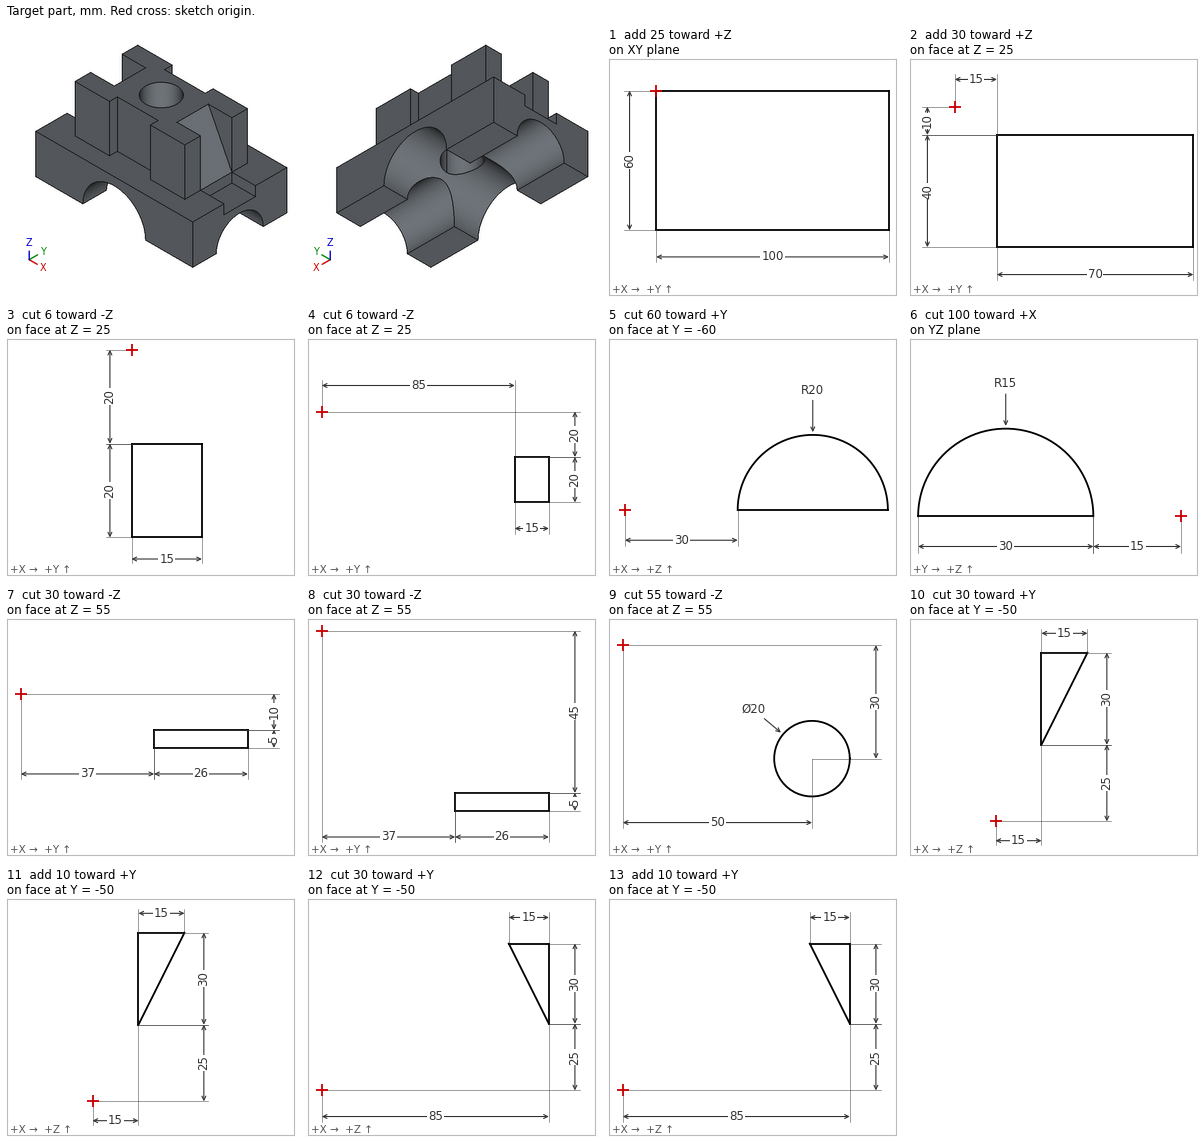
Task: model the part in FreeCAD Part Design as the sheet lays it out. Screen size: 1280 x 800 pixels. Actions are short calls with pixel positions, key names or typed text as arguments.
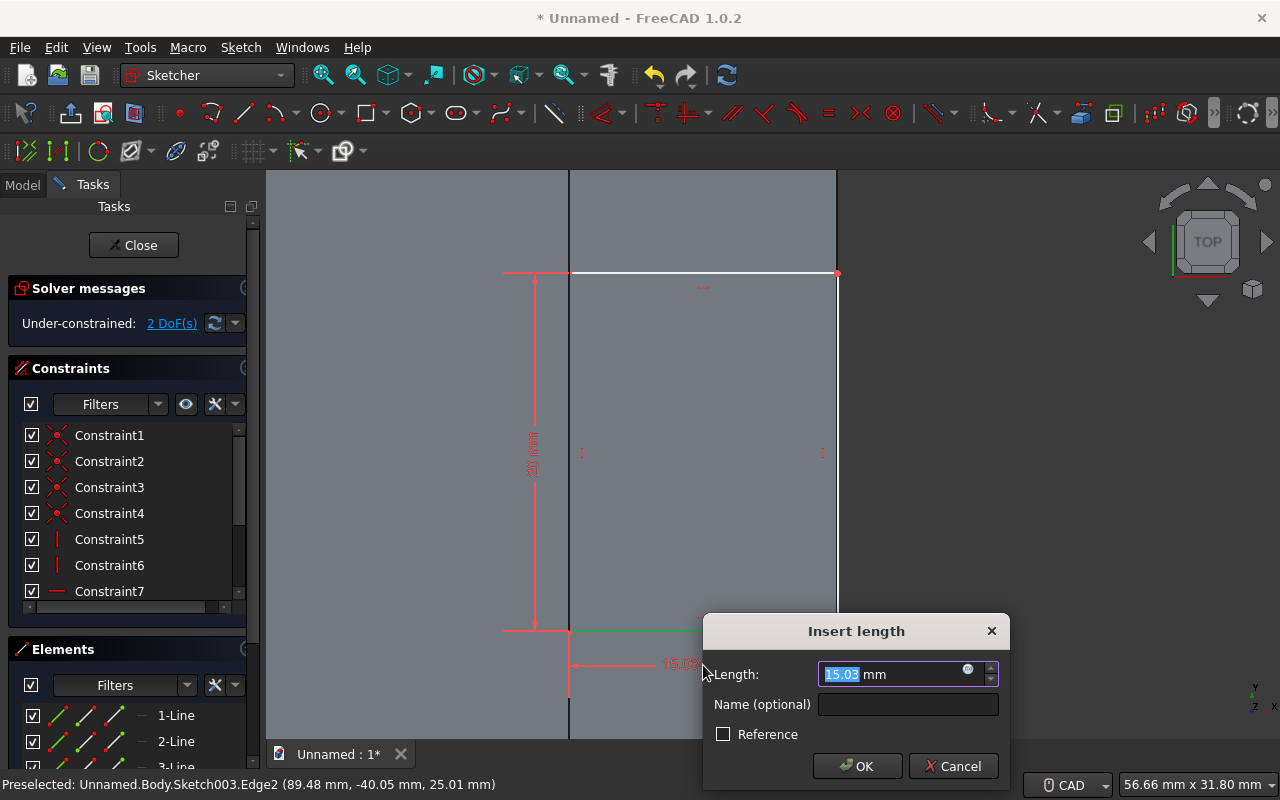
text(15)
key(Return)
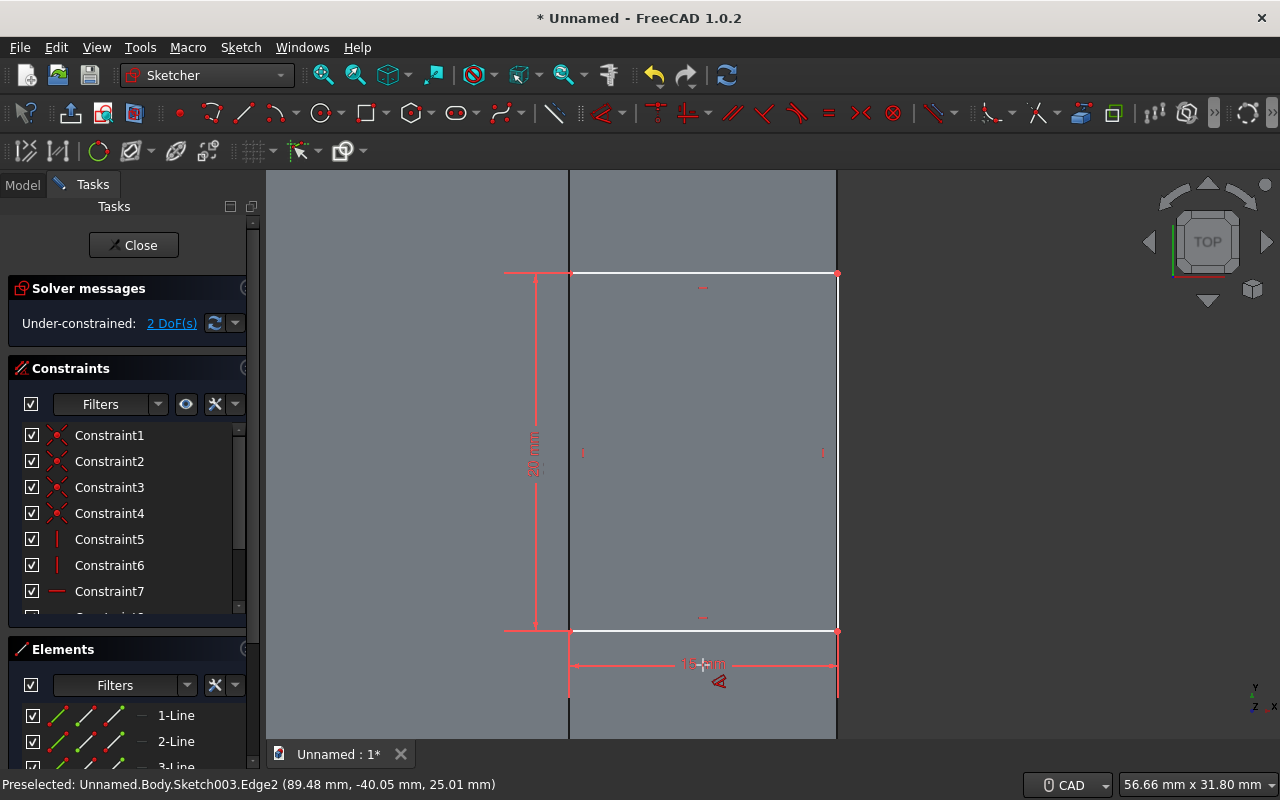
click(569, 273)
click(432, 307)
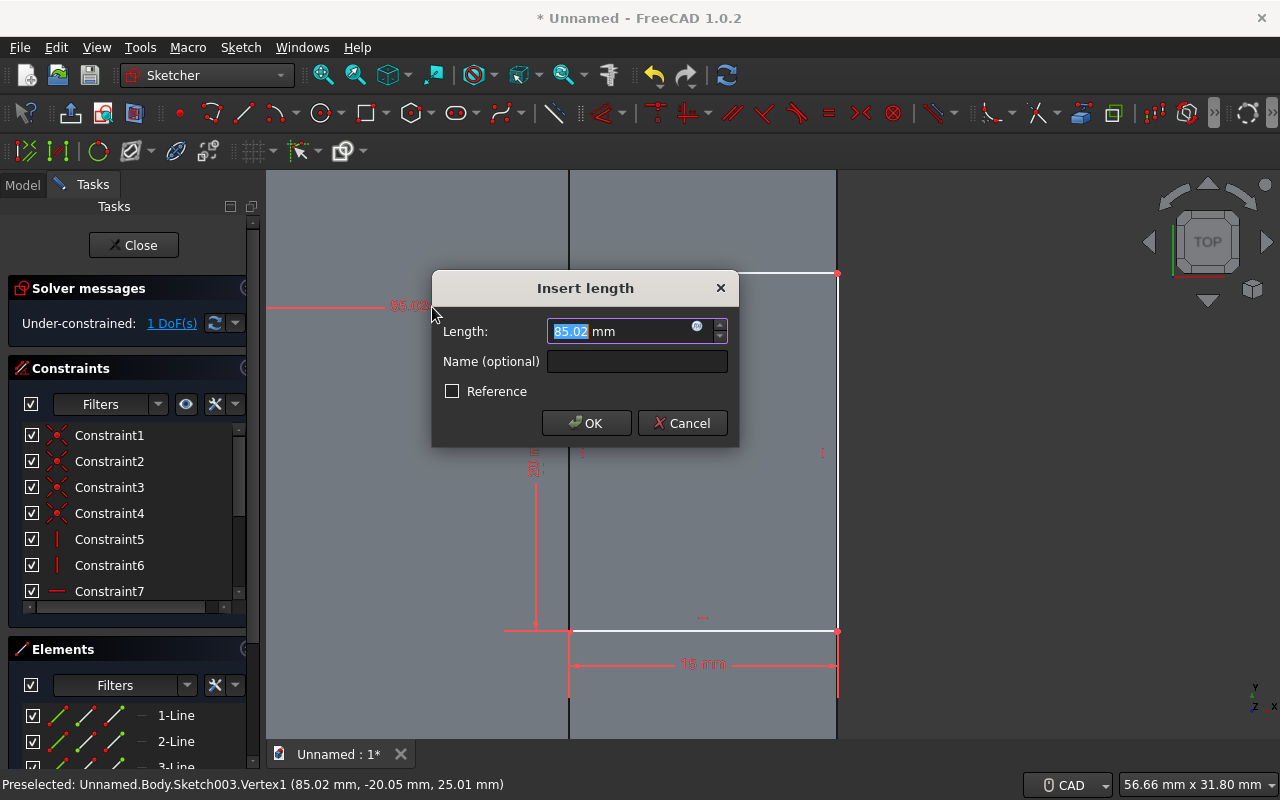
text(85)
key(Return)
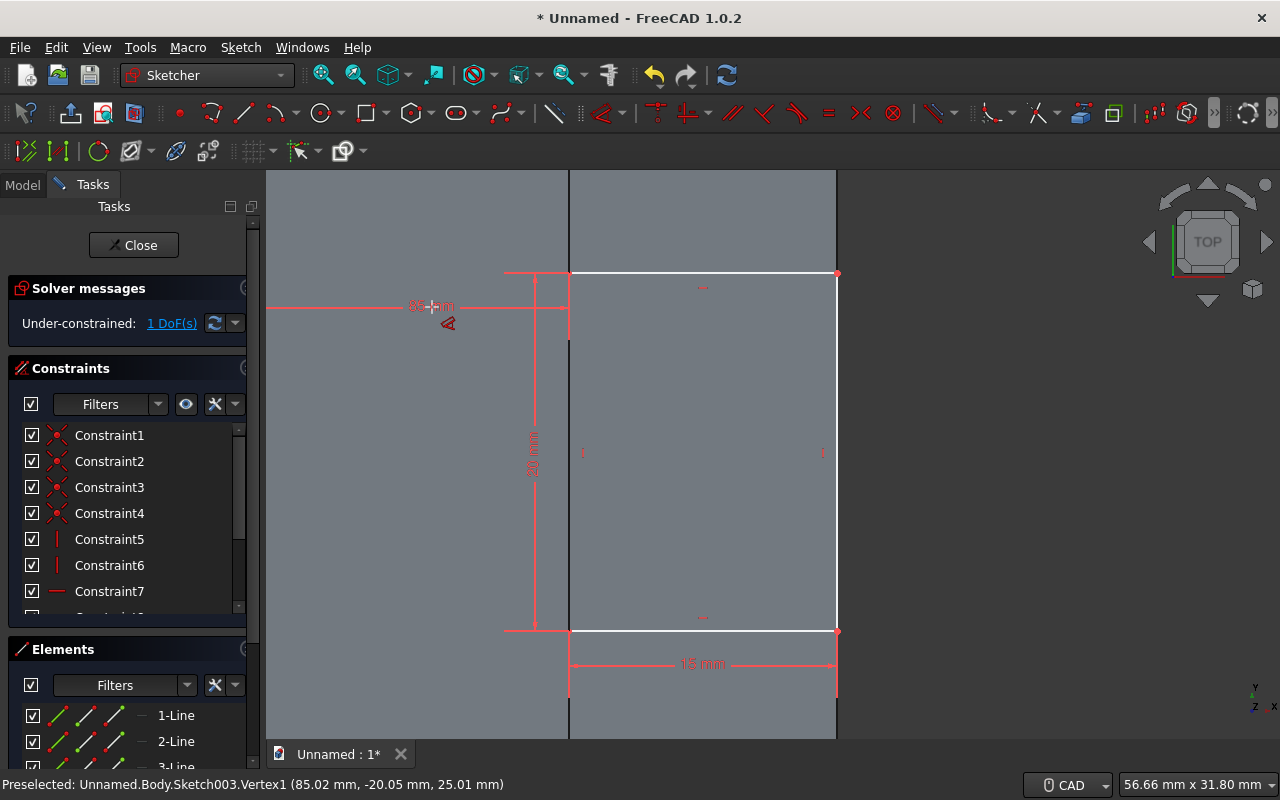
click(569, 273)
click(603, 236)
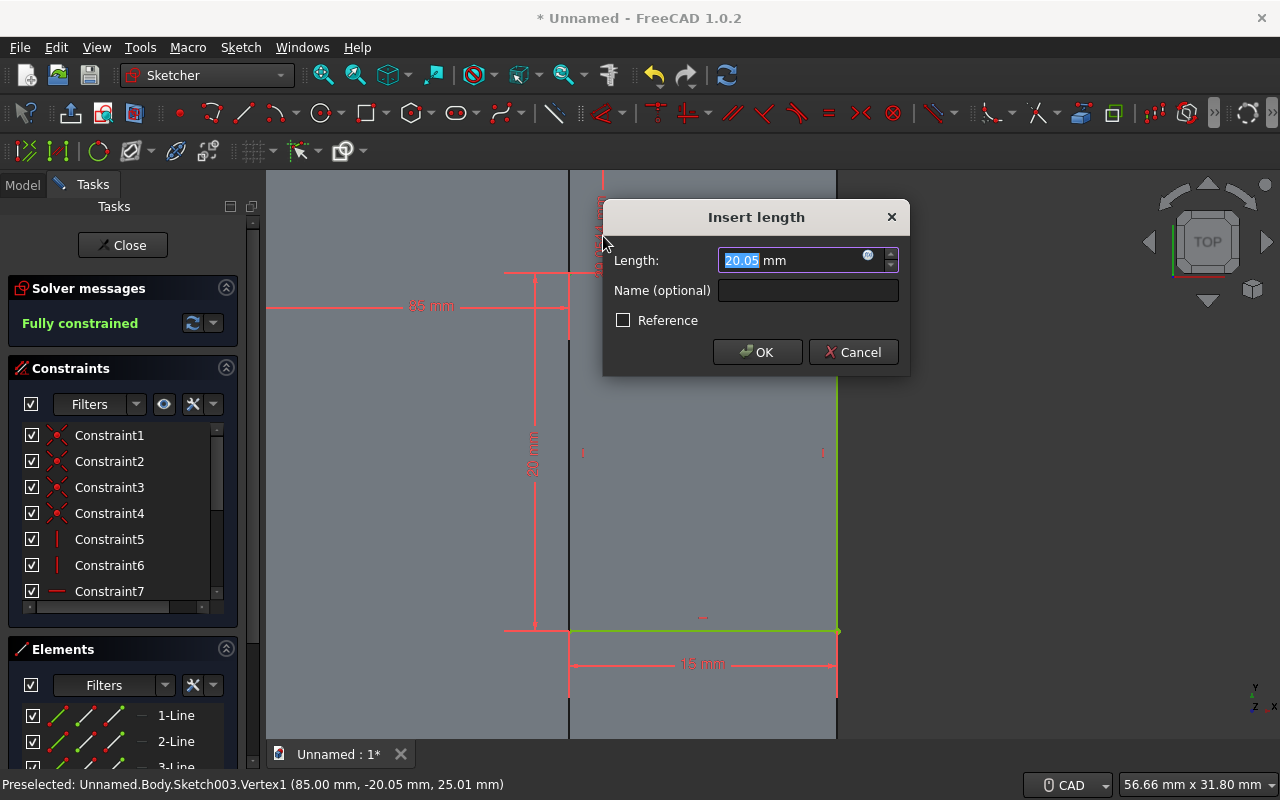
text(20)
key(Return)
key(Escape)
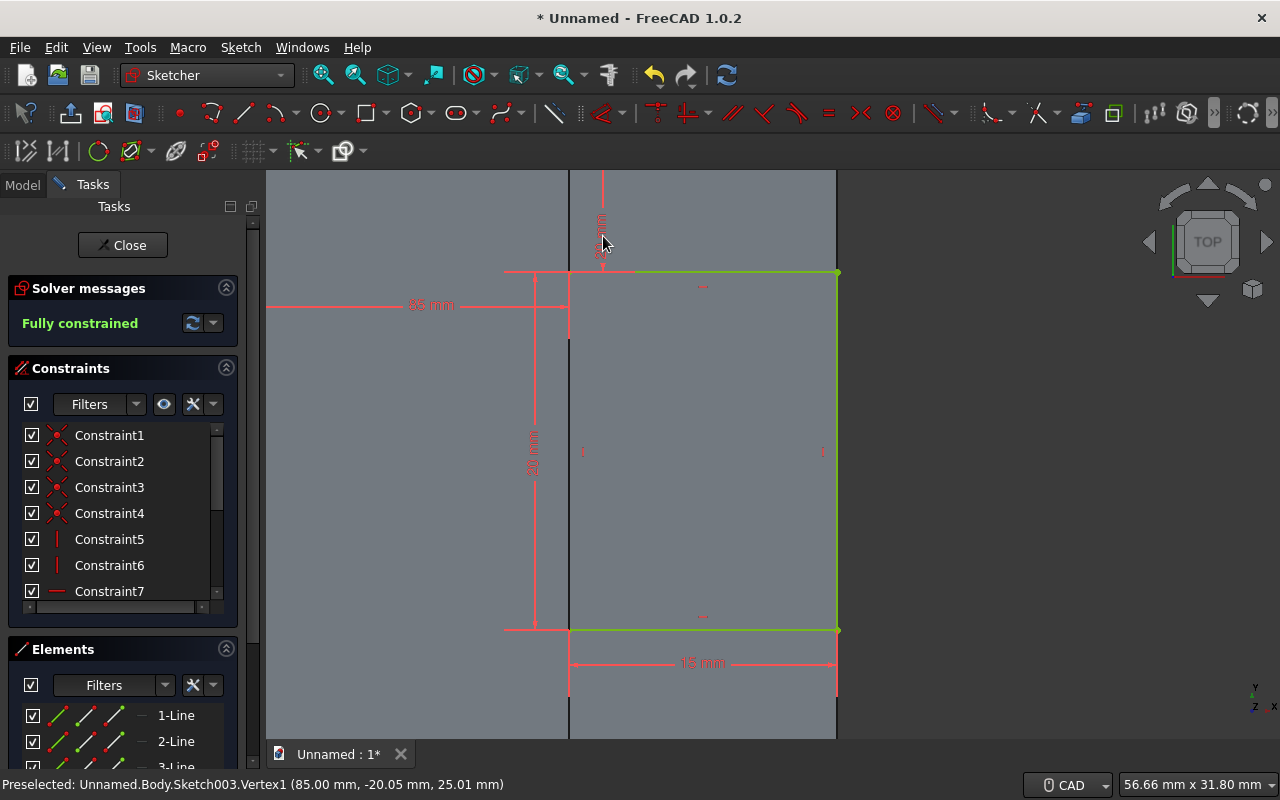
click(123, 245)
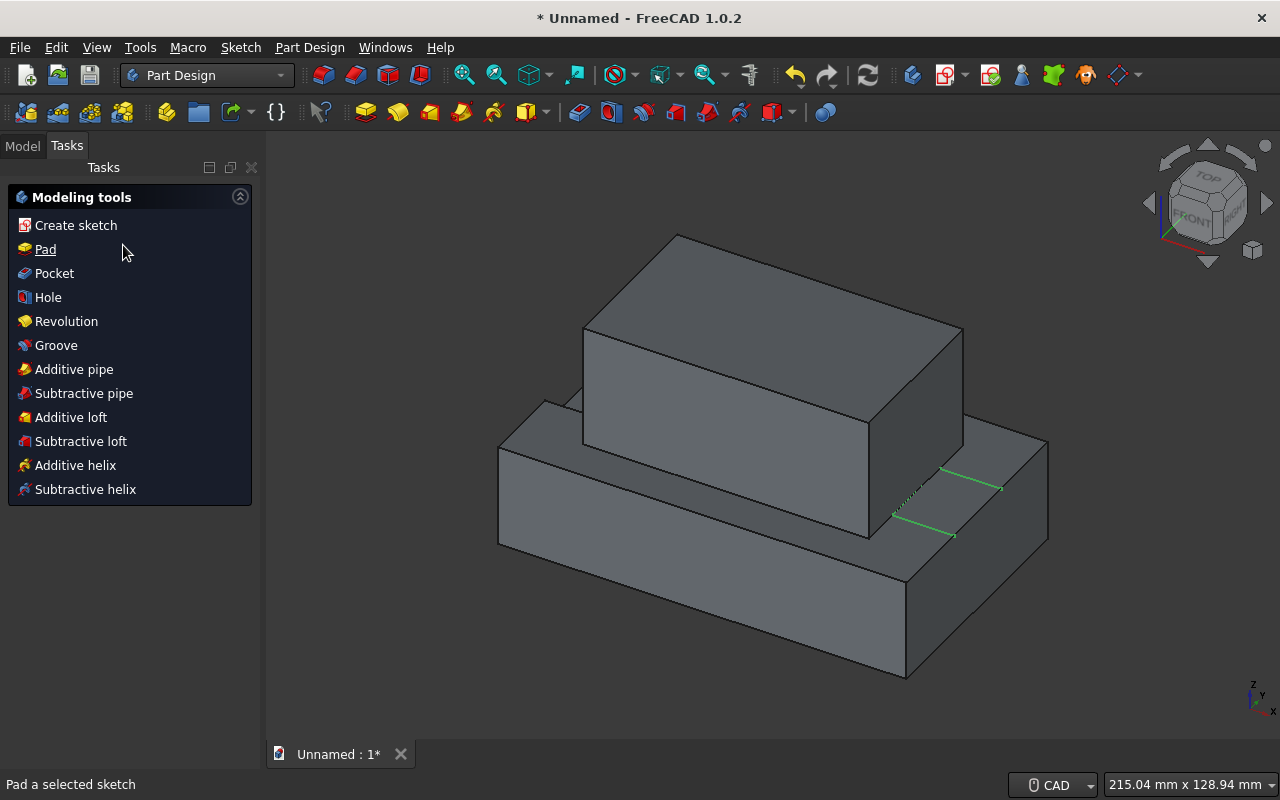
click(580, 112)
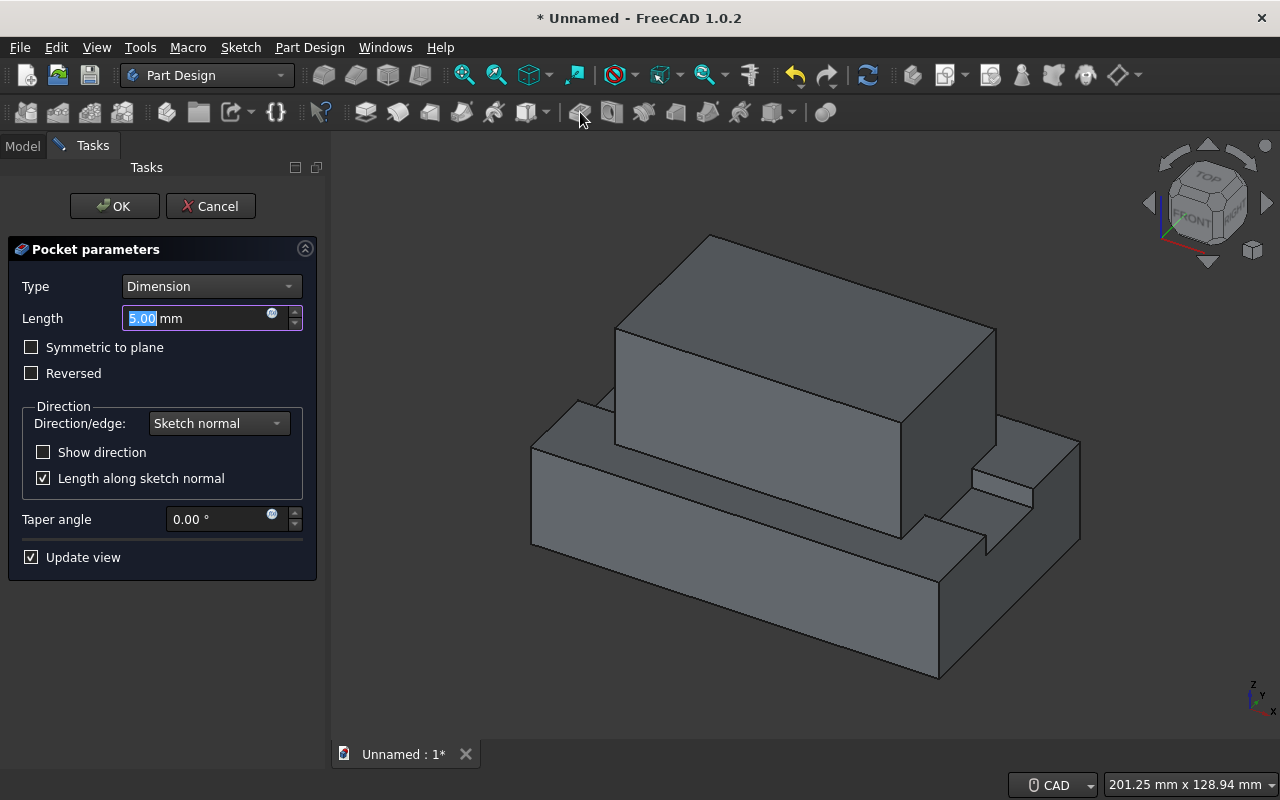
text(6)
key(Tab)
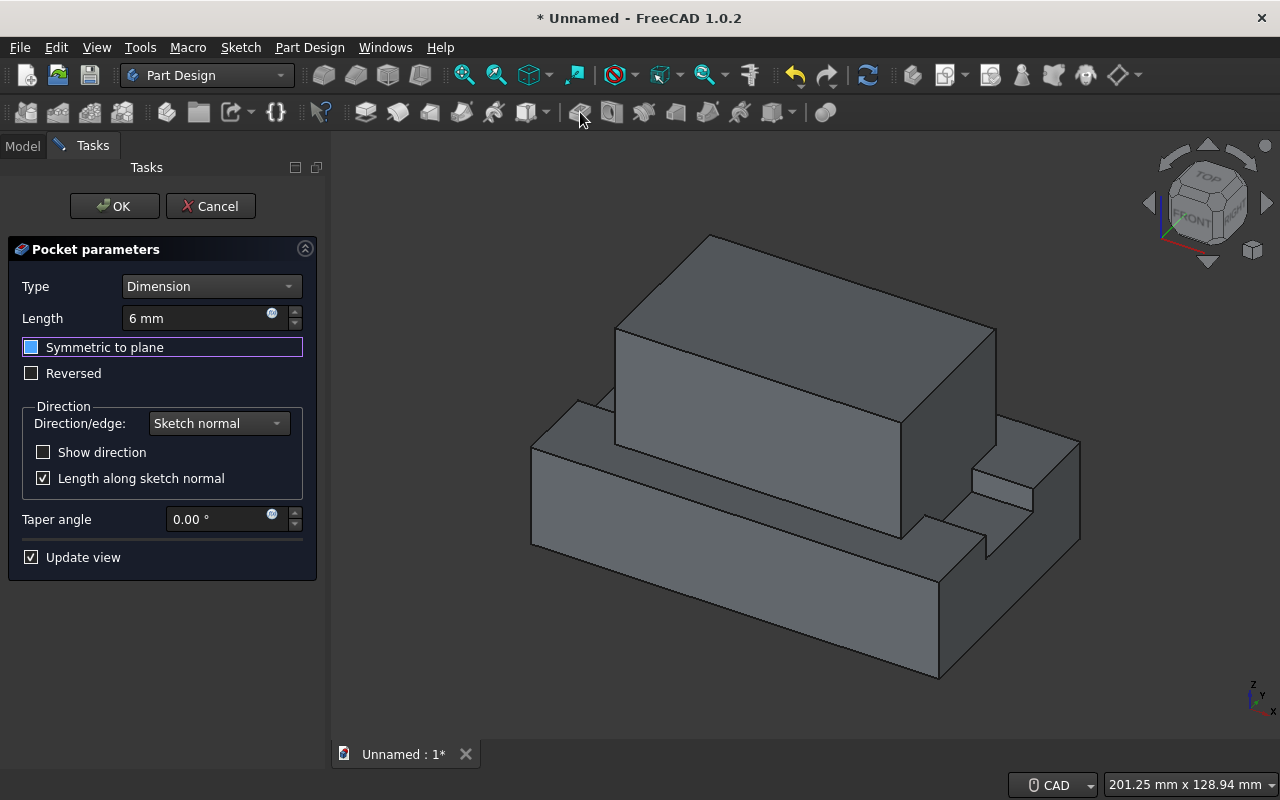
click(115, 206)